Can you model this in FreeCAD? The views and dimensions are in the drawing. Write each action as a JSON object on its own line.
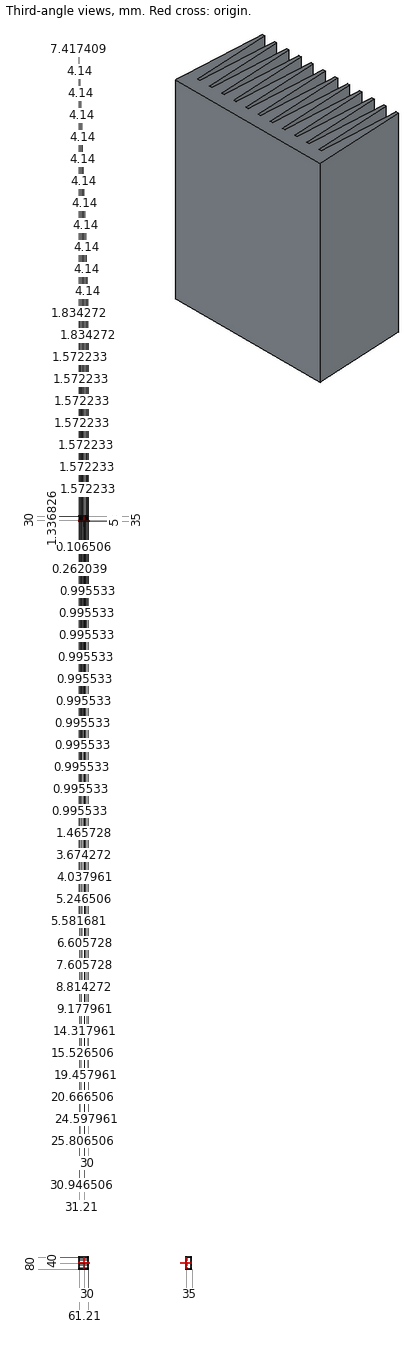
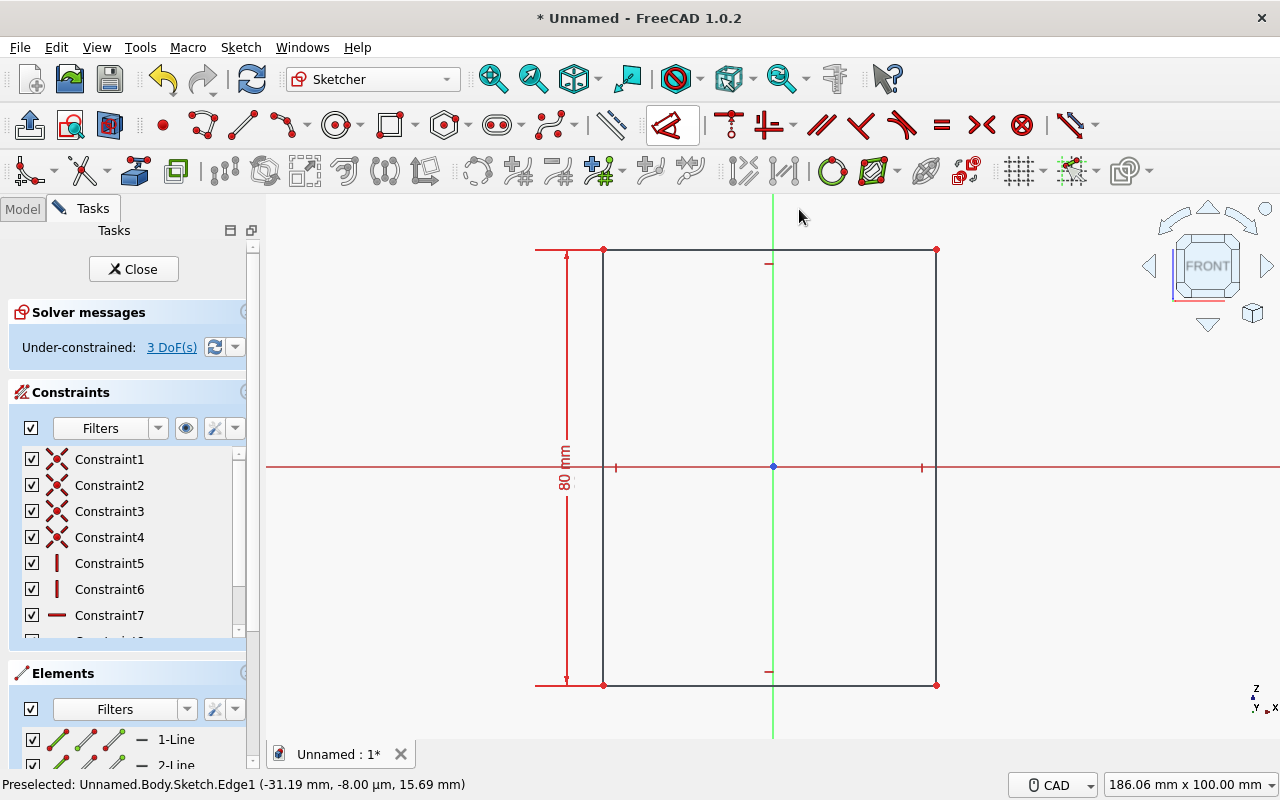
{"action": "left_click", "coordinate": [603, 250]}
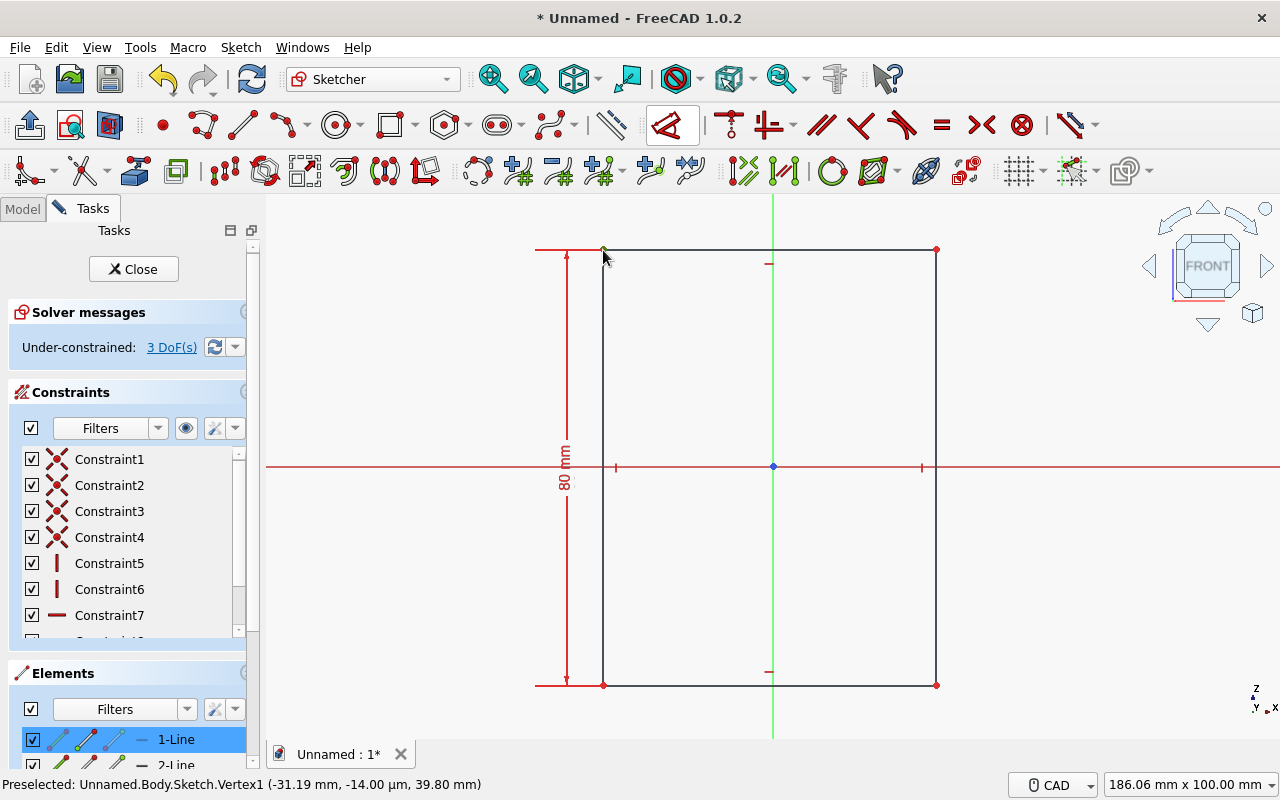
{"action": "left_click", "coordinate": [694, 126]}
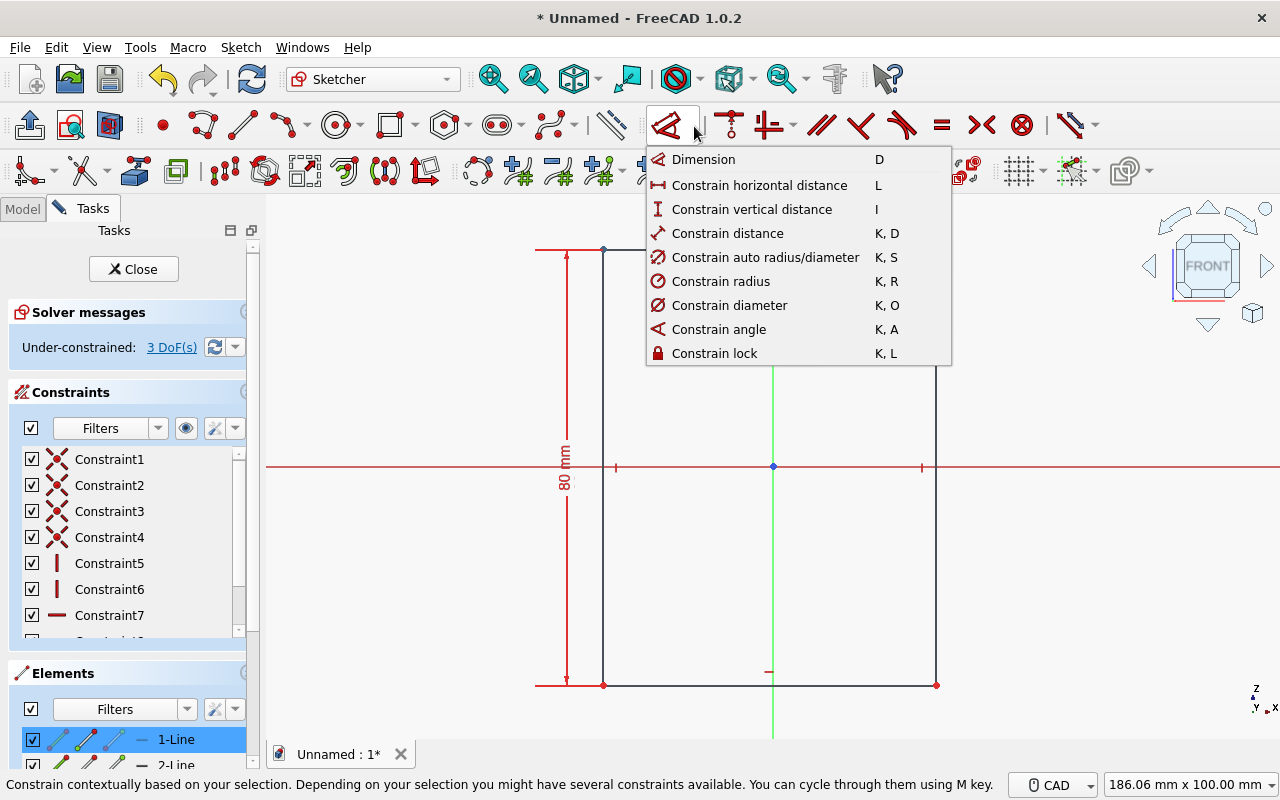
{"action": "left_click", "coordinate": [799, 209]}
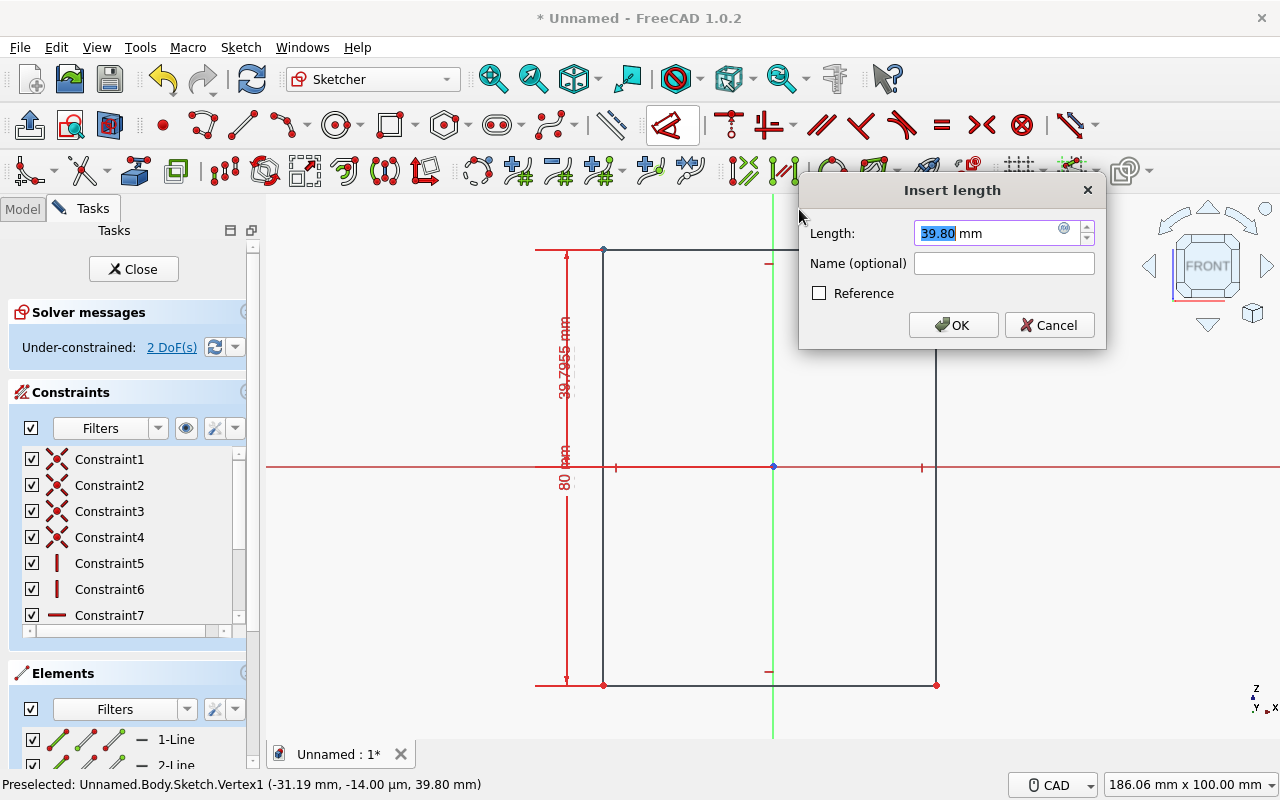
{"action": "type", "text": "40"}
{"action": "key", "text": "Return"}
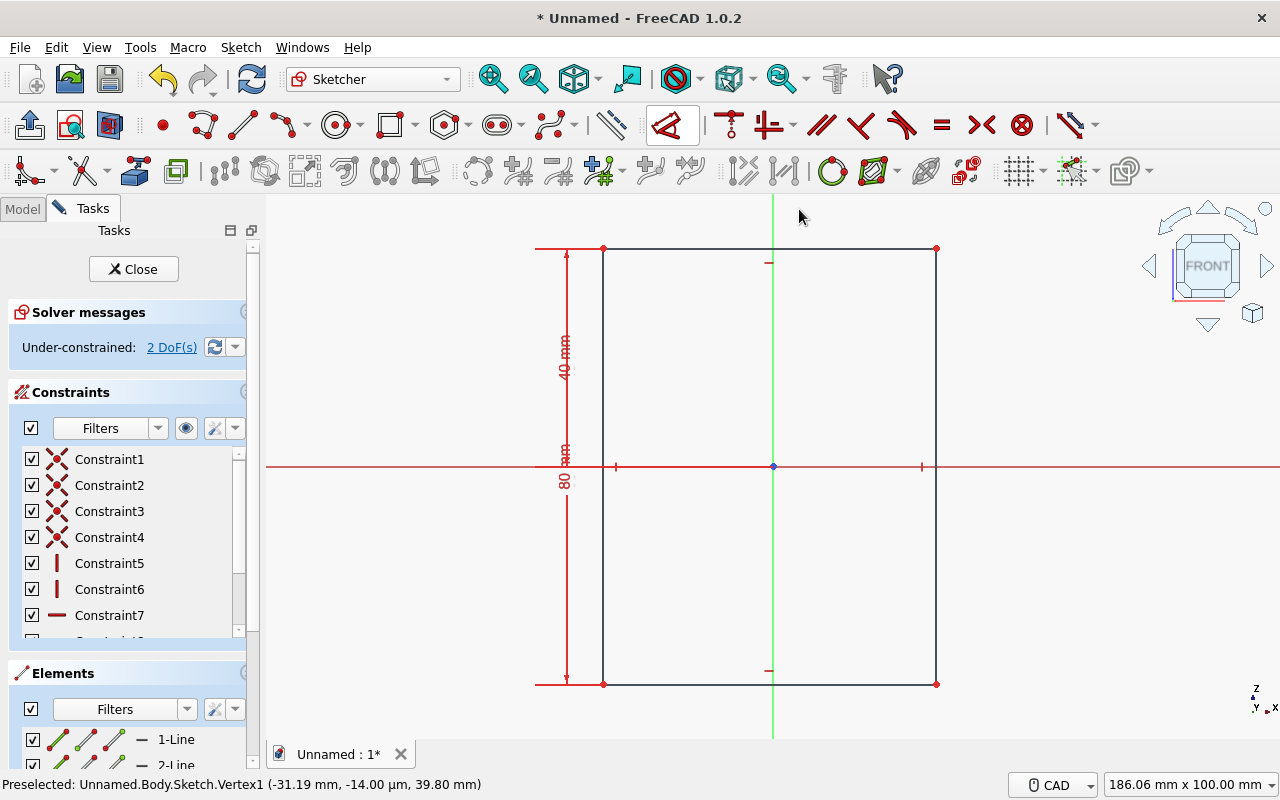
{"action": "left_click", "coordinate": [936, 684]}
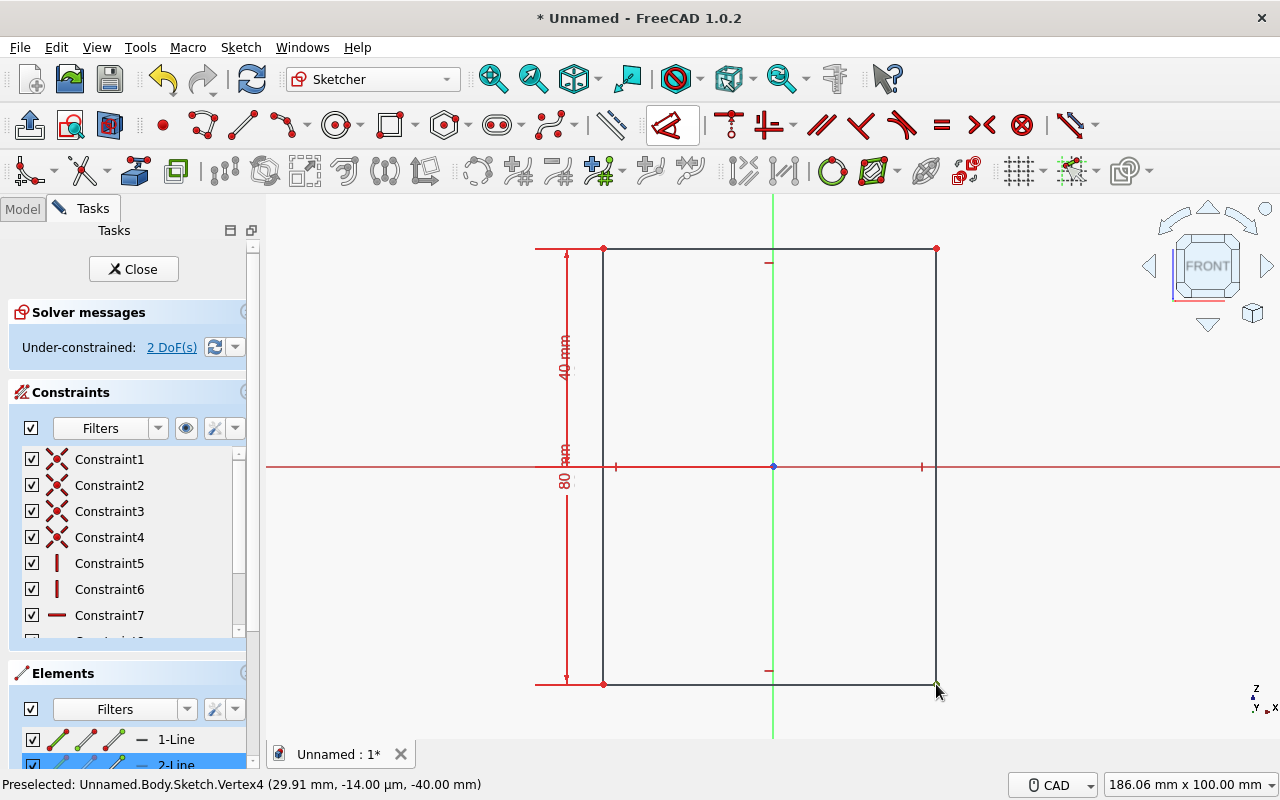
{"action": "key", "text": "l"}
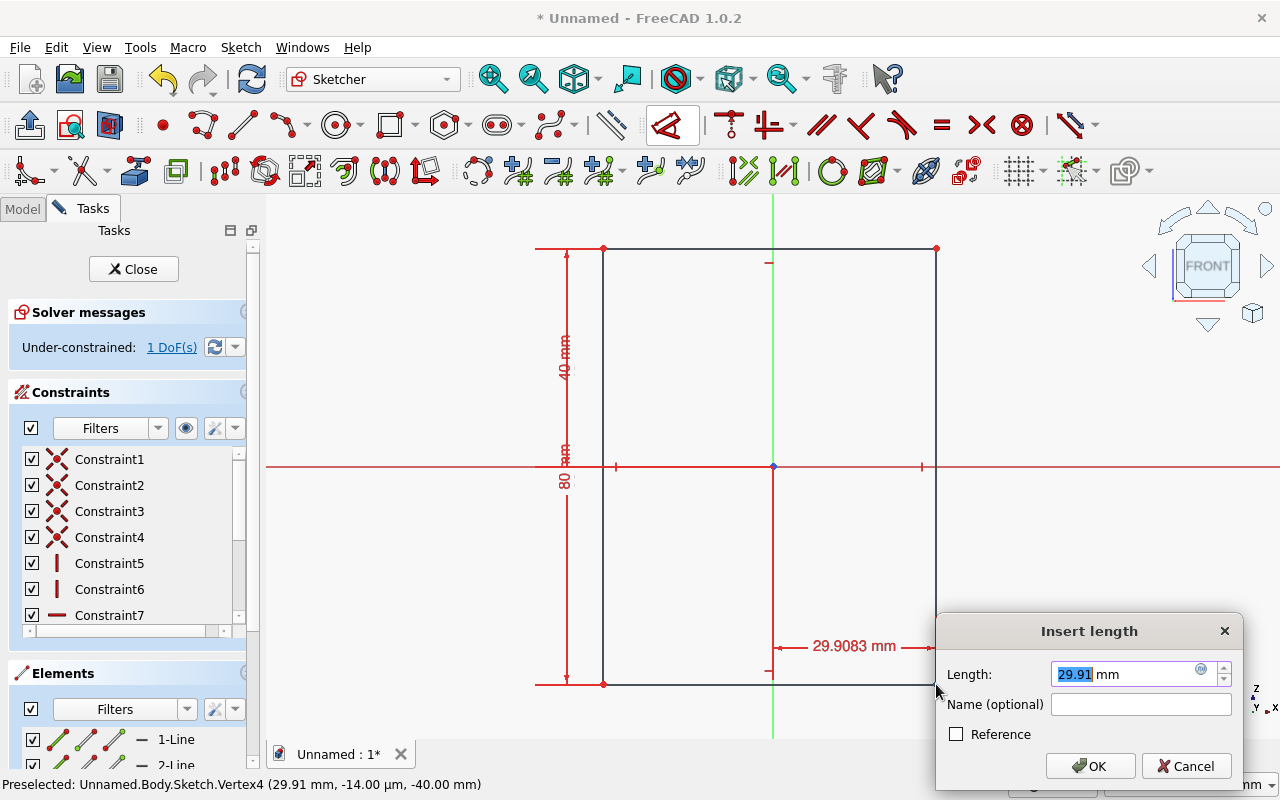
{"action": "type", "text": "30"}
{"action": "key", "text": "Return"}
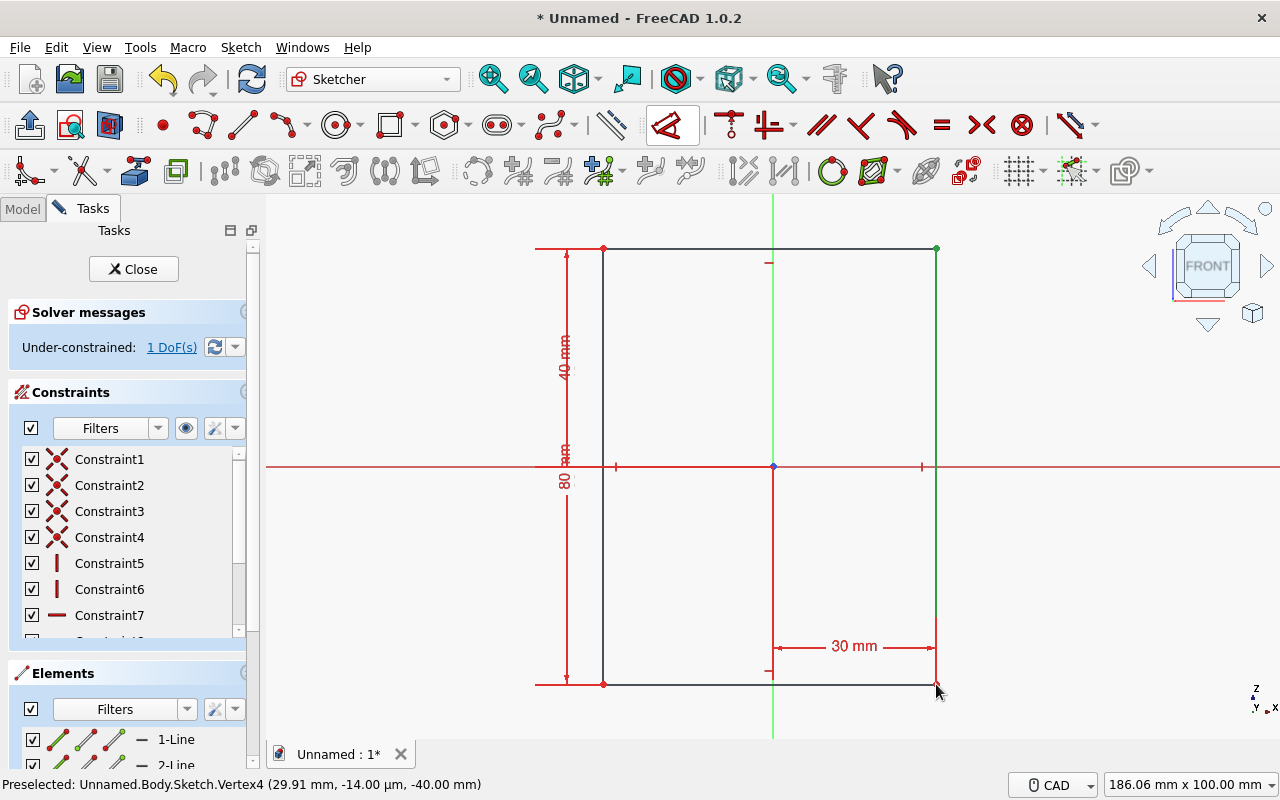
{"action": "left_click", "coordinate": [703, 684]}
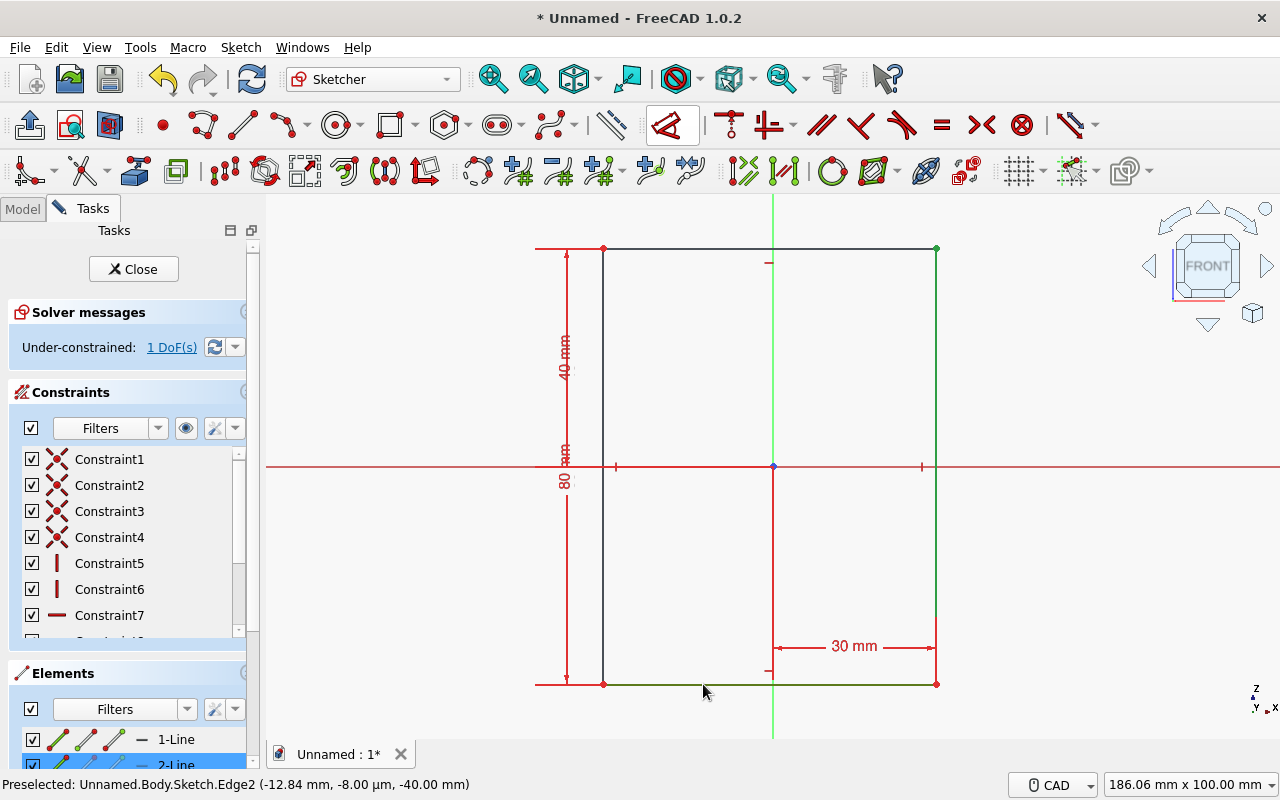
{"action": "left_click", "coordinate": [694, 126]}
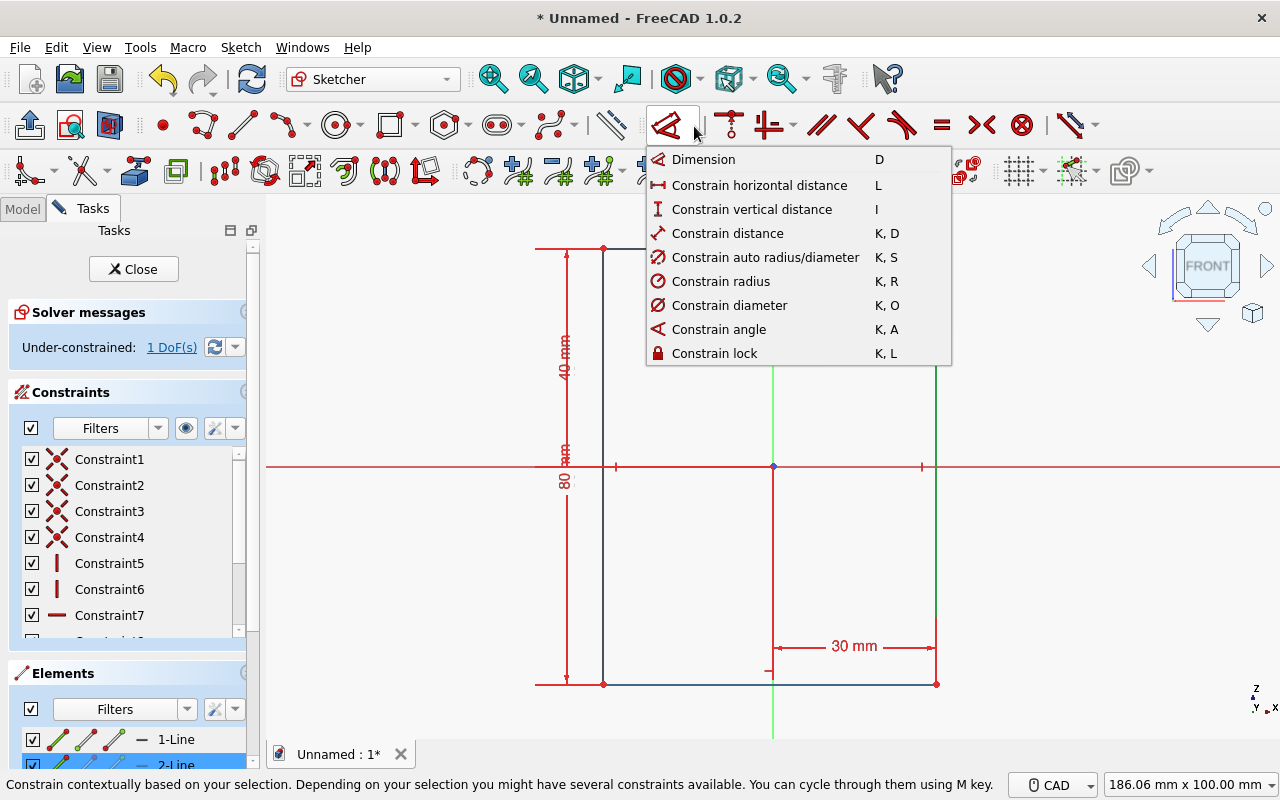
{"action": "left_click", "coordinate": [799, 185]}